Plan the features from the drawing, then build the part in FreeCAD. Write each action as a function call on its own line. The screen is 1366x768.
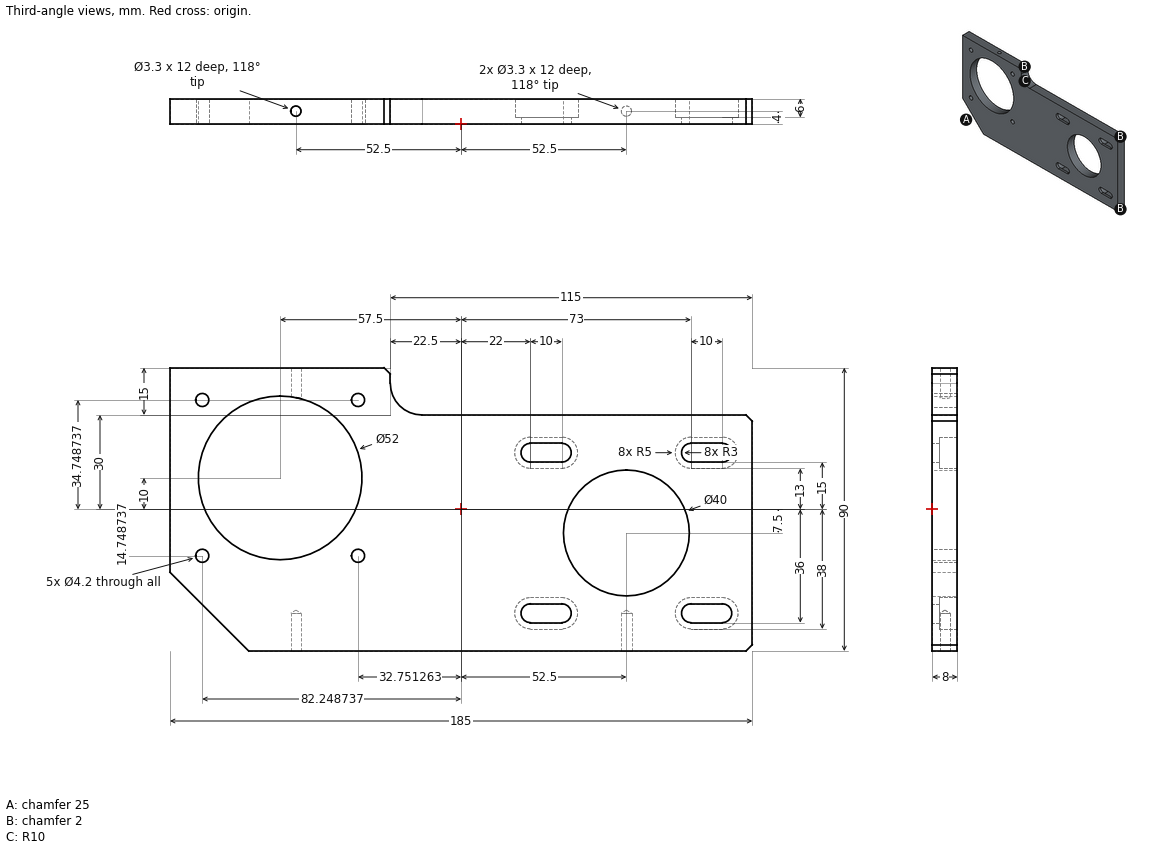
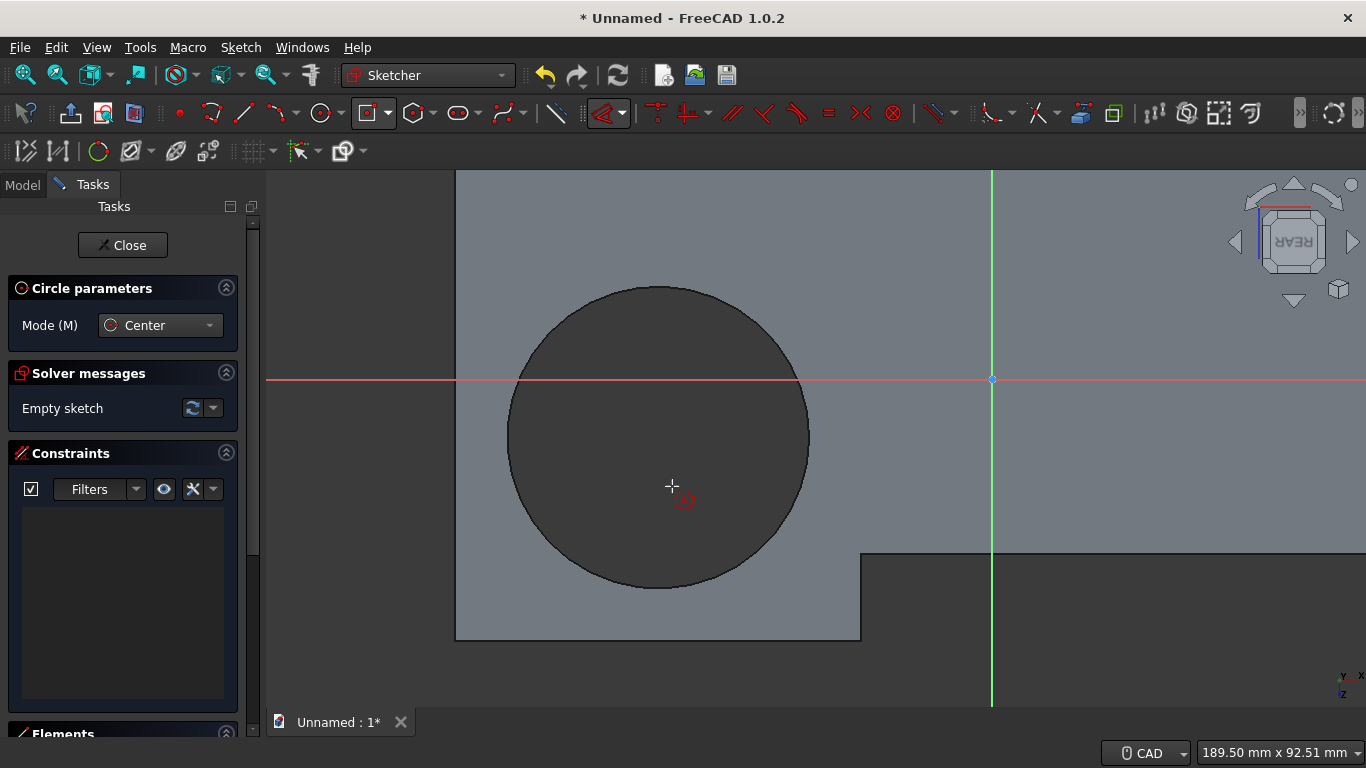
scroll(515, 294, up, 4)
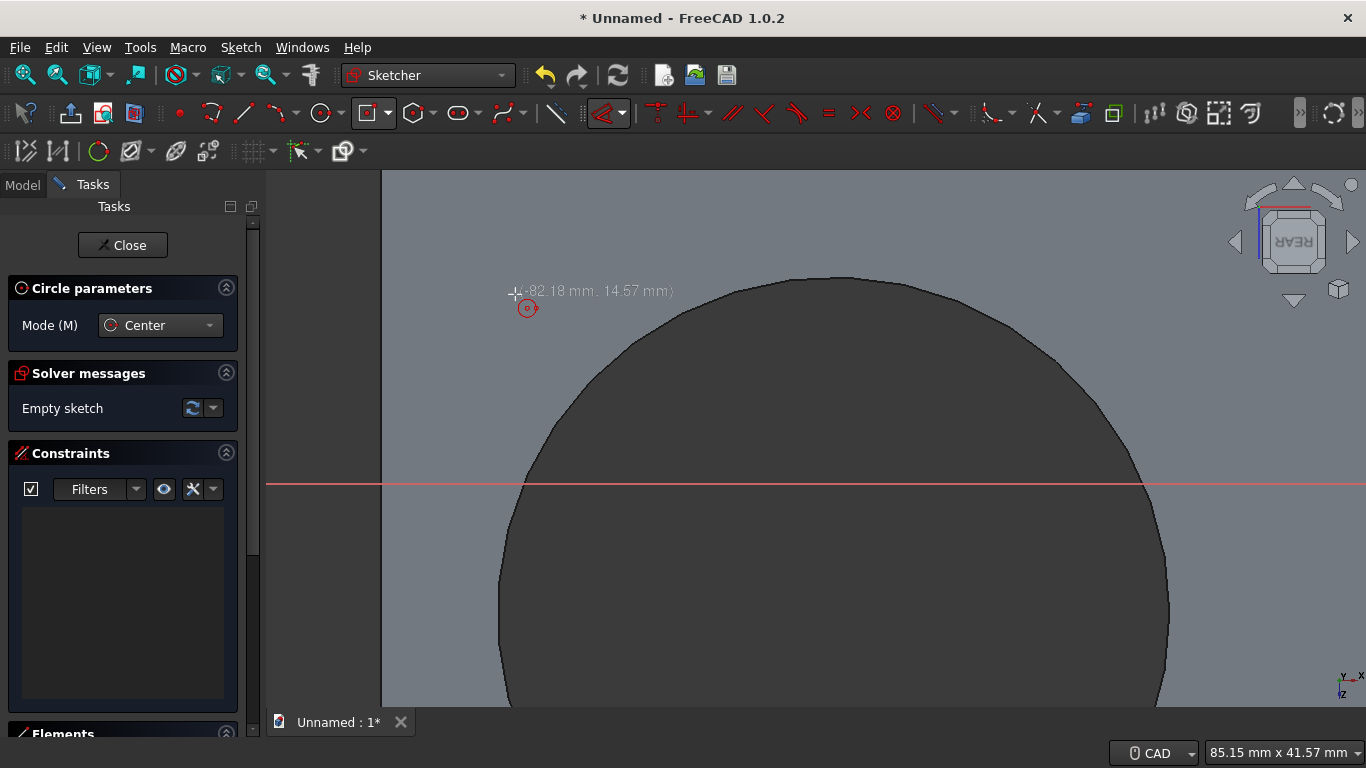
click(514, 294)
click(533, 274)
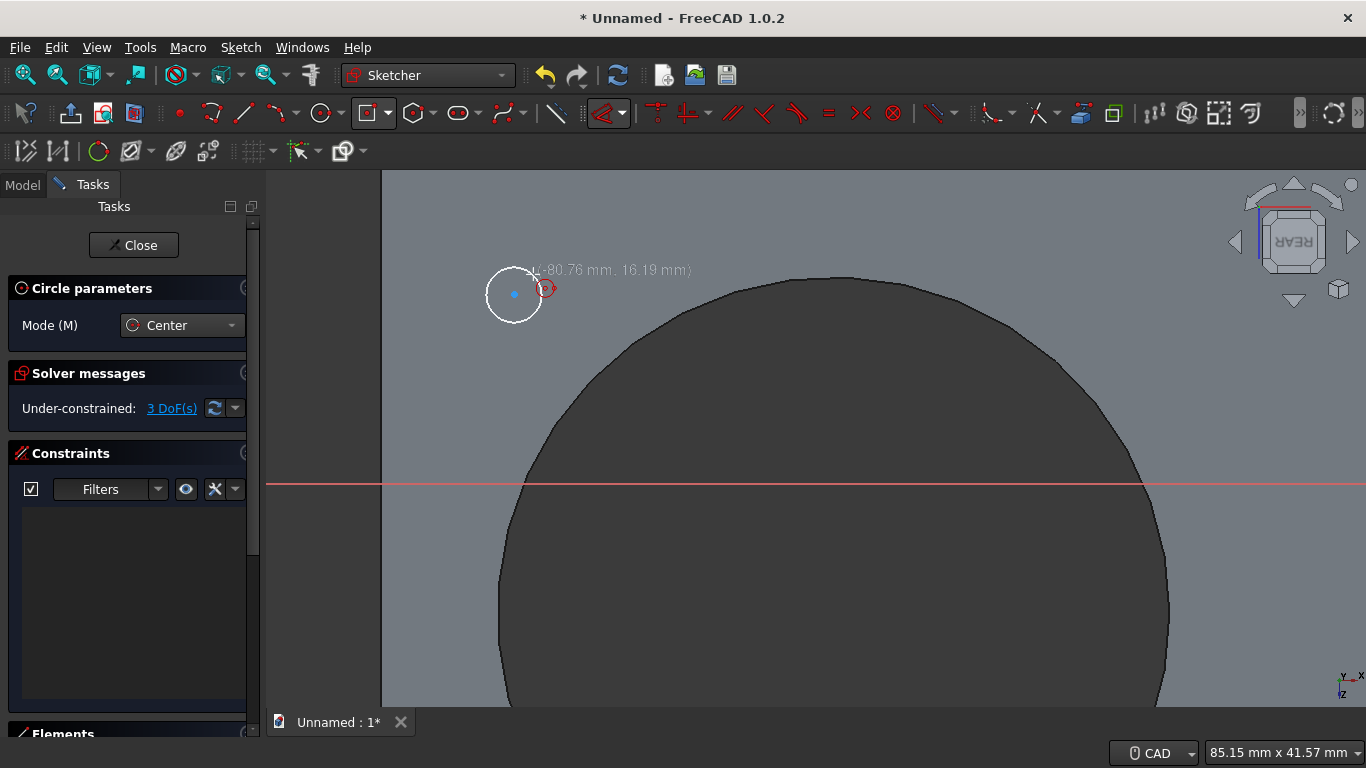
click(1153, 294)
click(1172, 274)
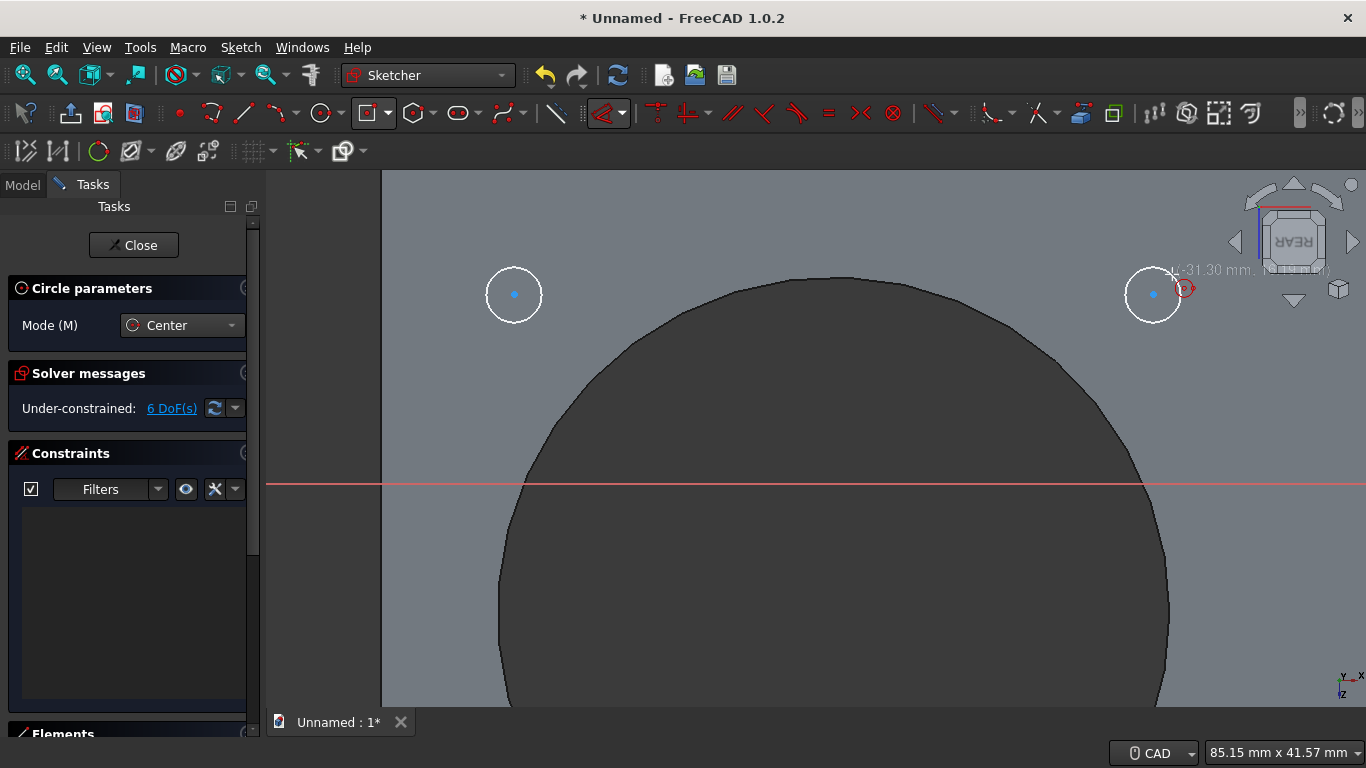
scroll(516, 296, down, 4)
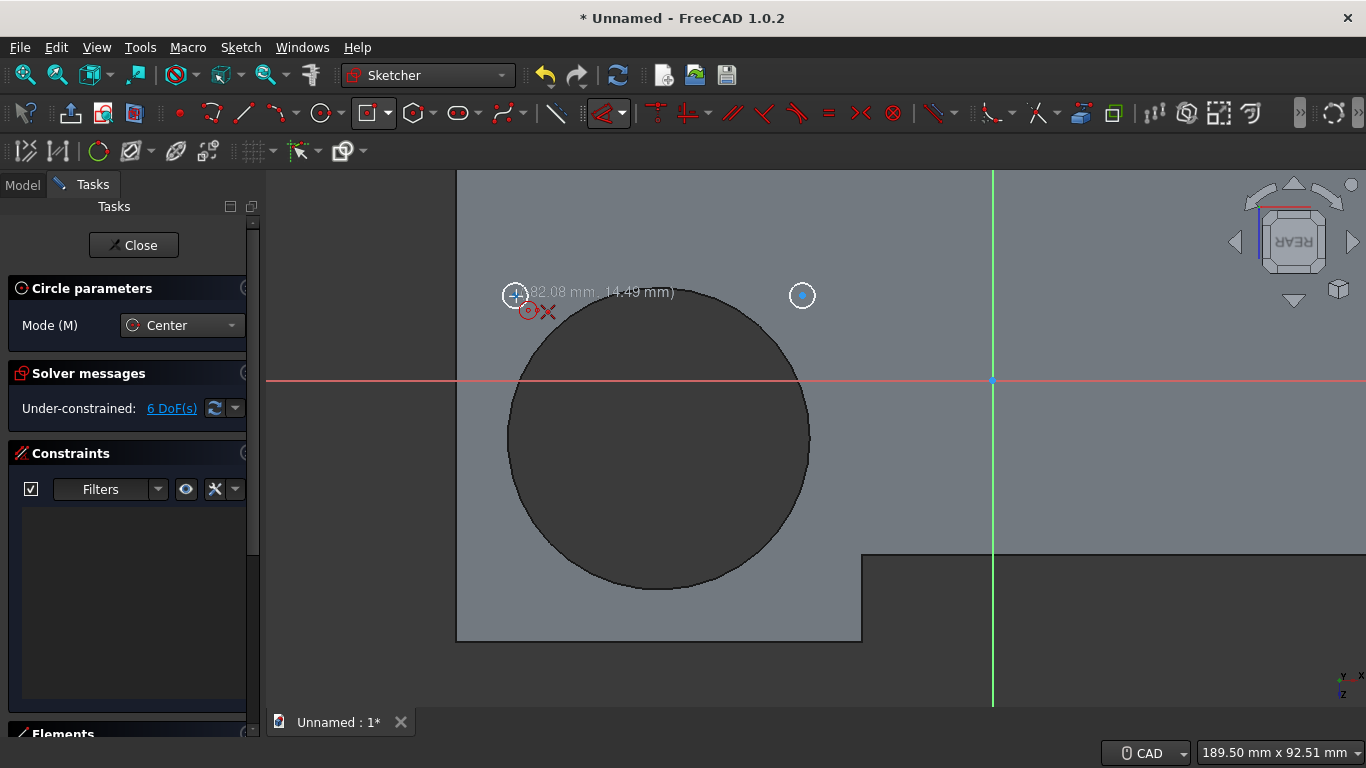
scroll(802, 582, up, 4)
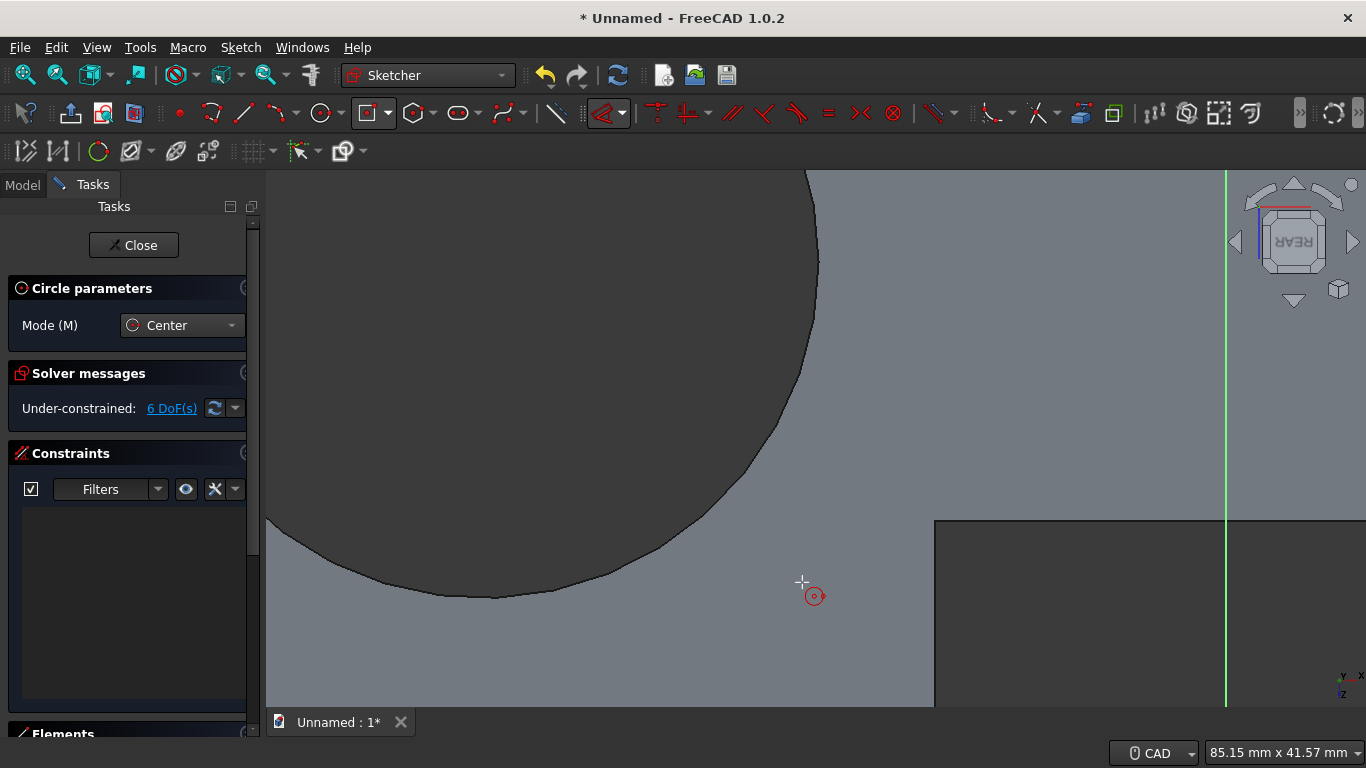
click(802, 582)
click(822, 563)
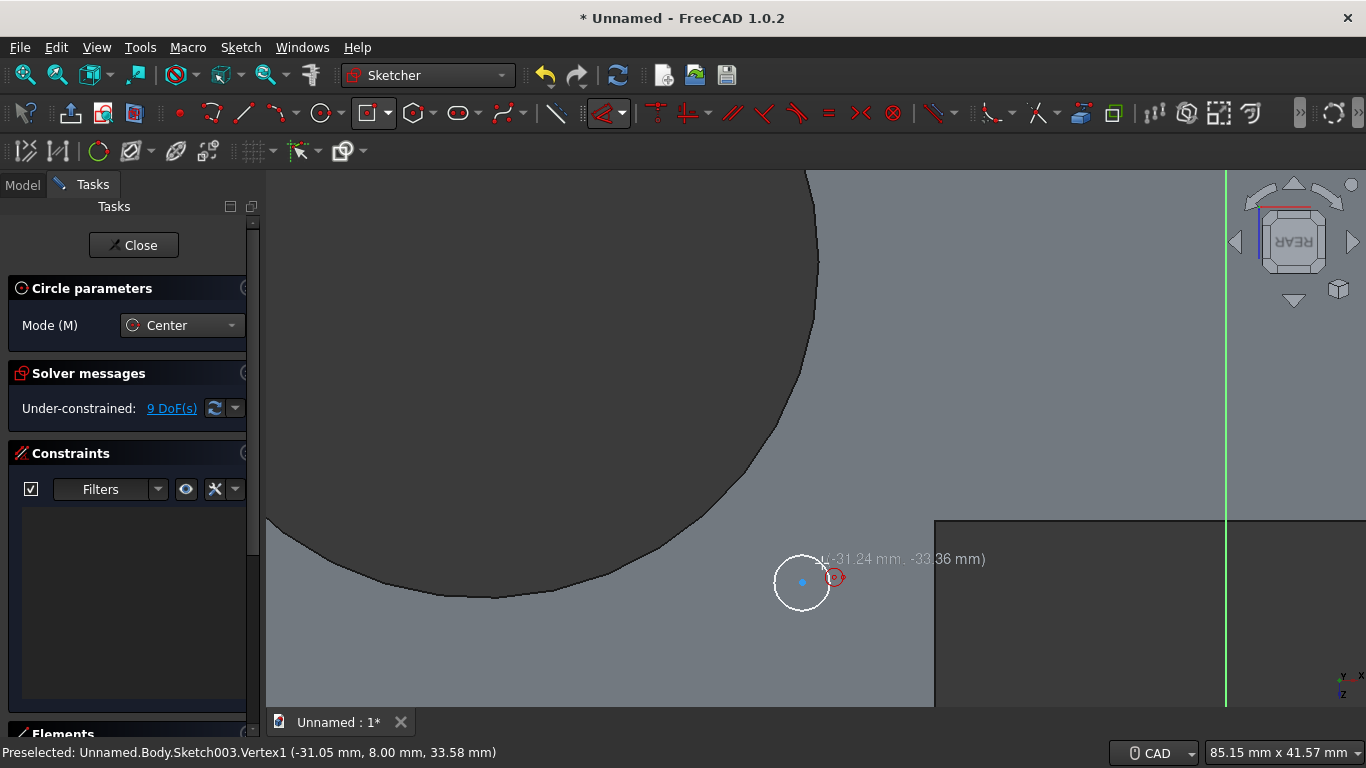
scroll(802, 582, down, 4)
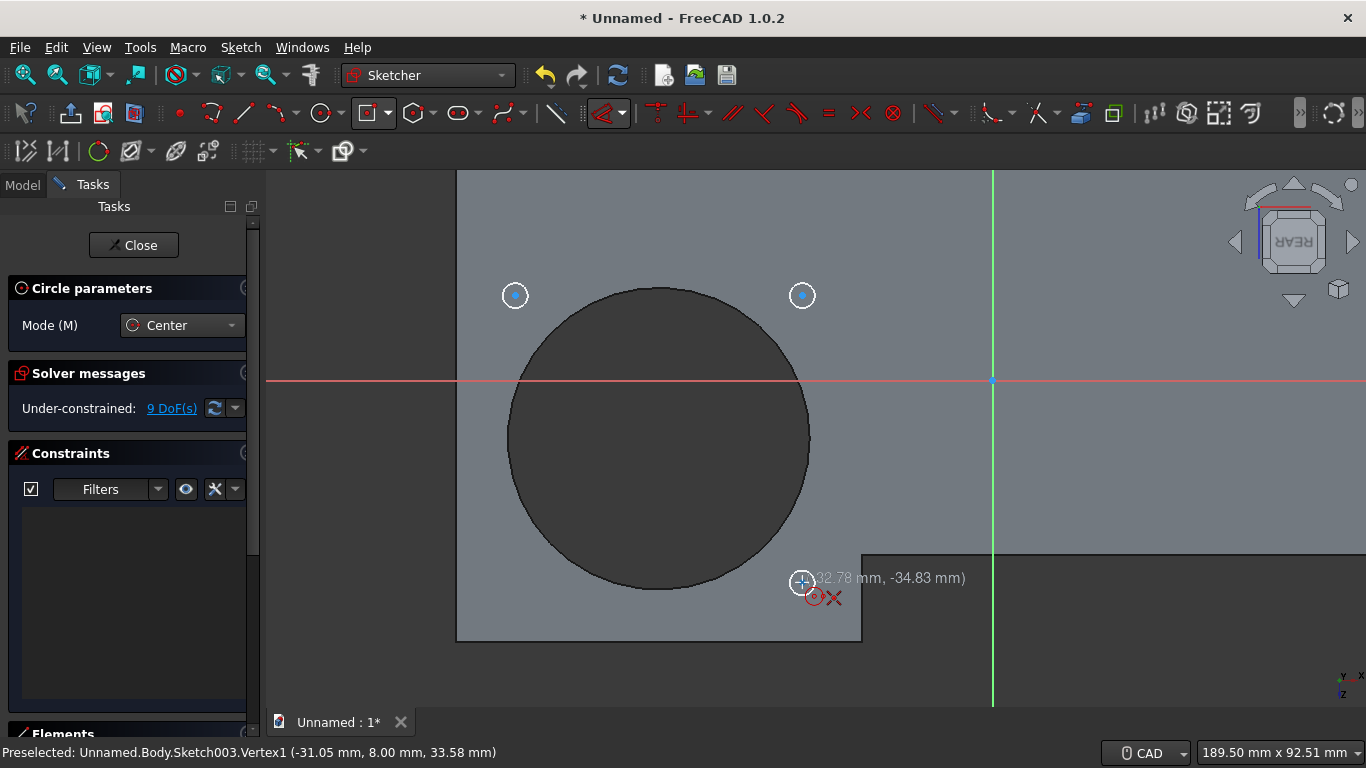
scroll(515, 582, up, 4)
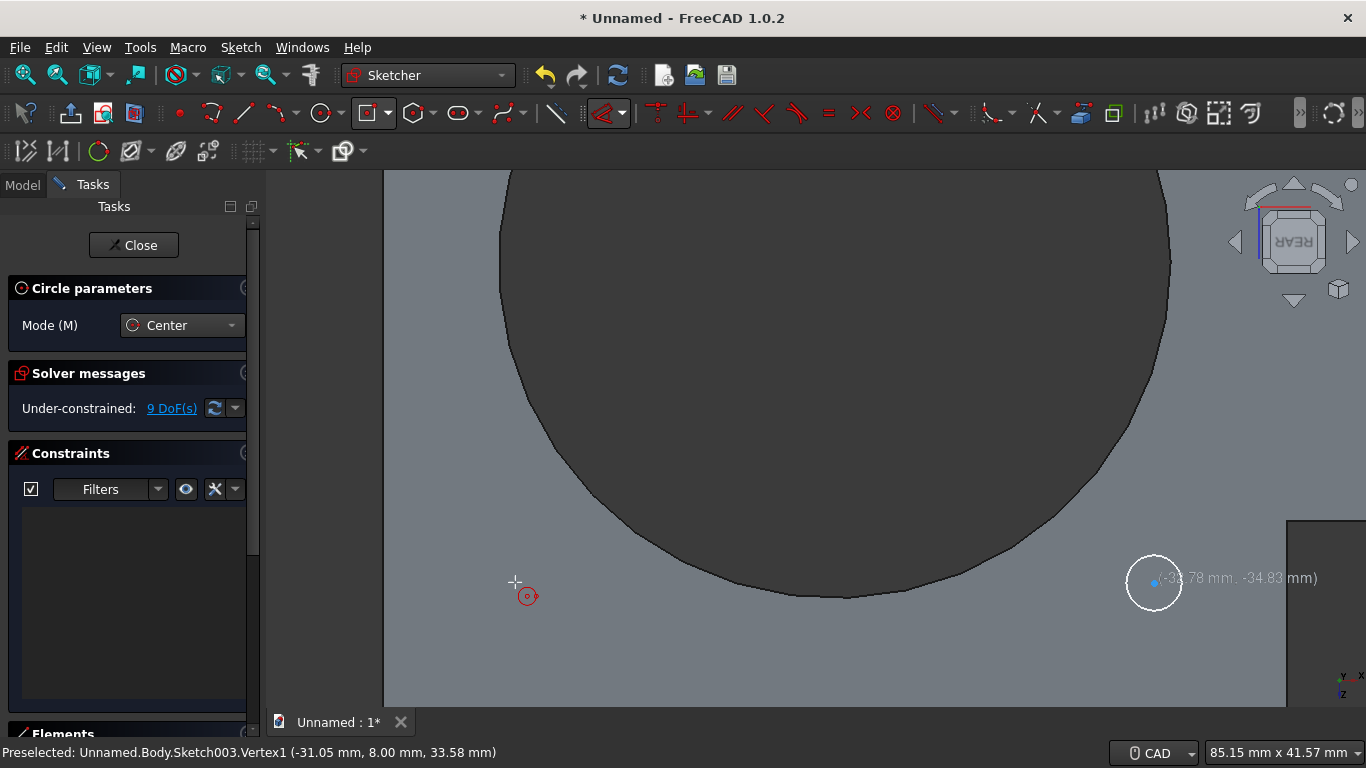
click(515, 582)
click(534, 563)